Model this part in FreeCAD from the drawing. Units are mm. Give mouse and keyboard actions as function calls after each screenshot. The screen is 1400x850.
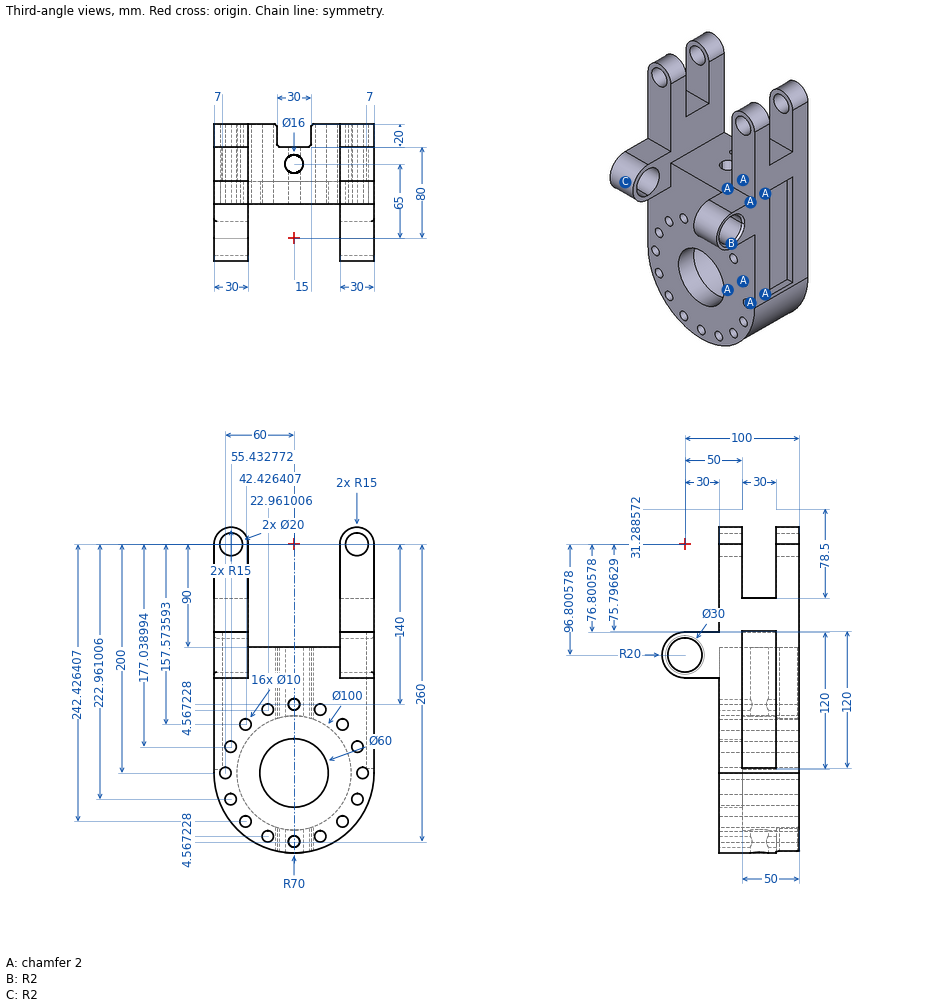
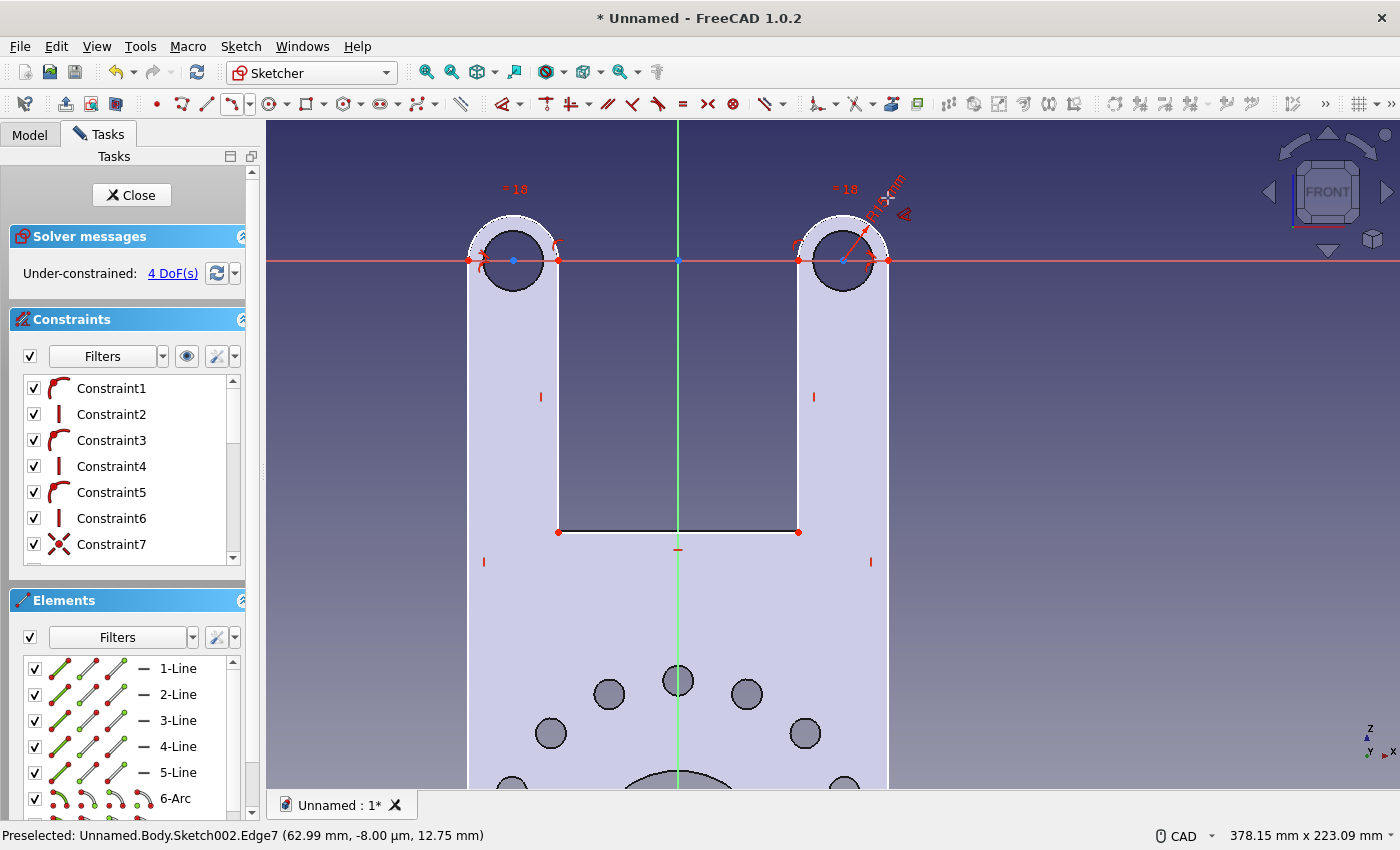
click(798, 342)
click(832, 397)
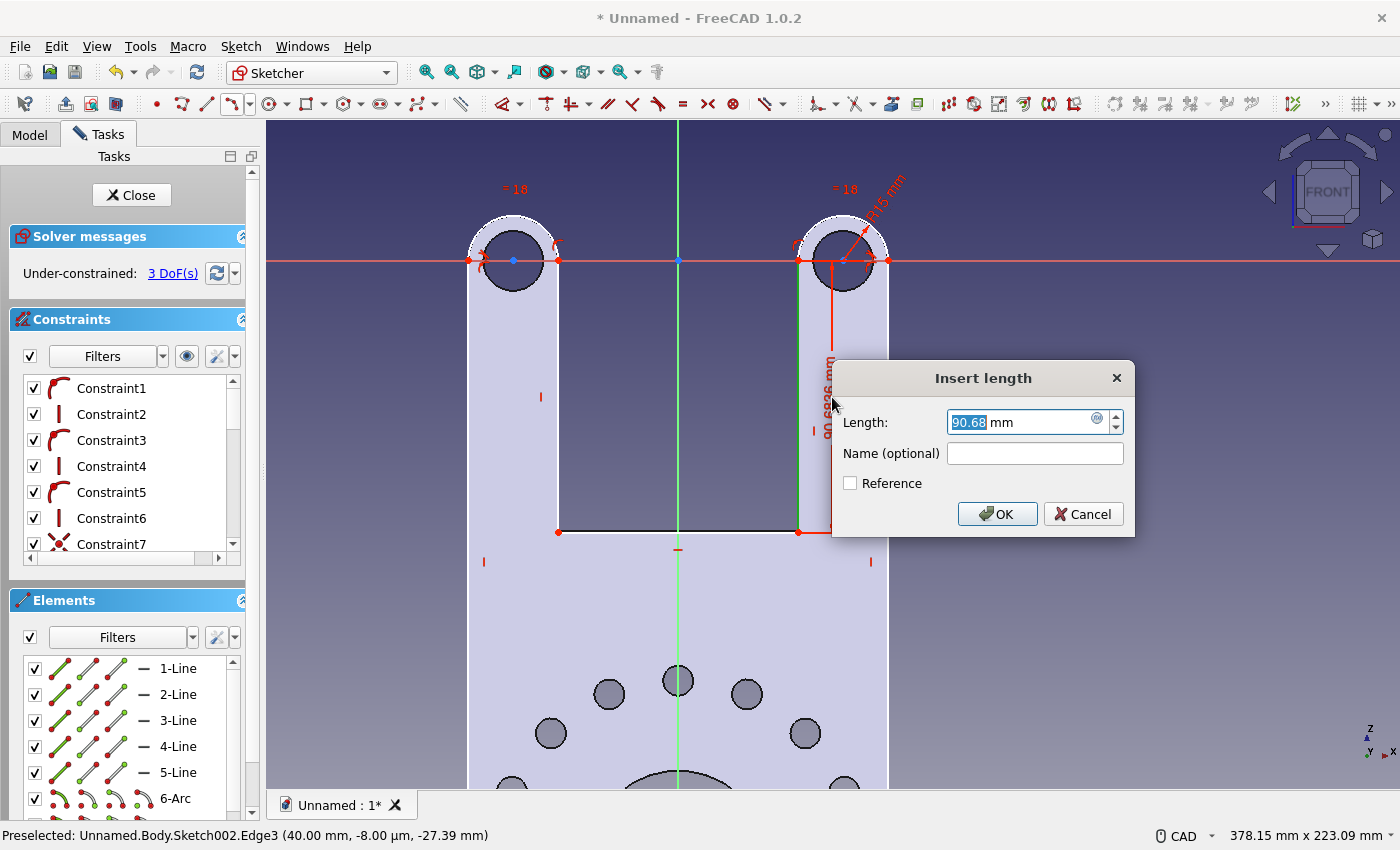
text(90)
key(Return)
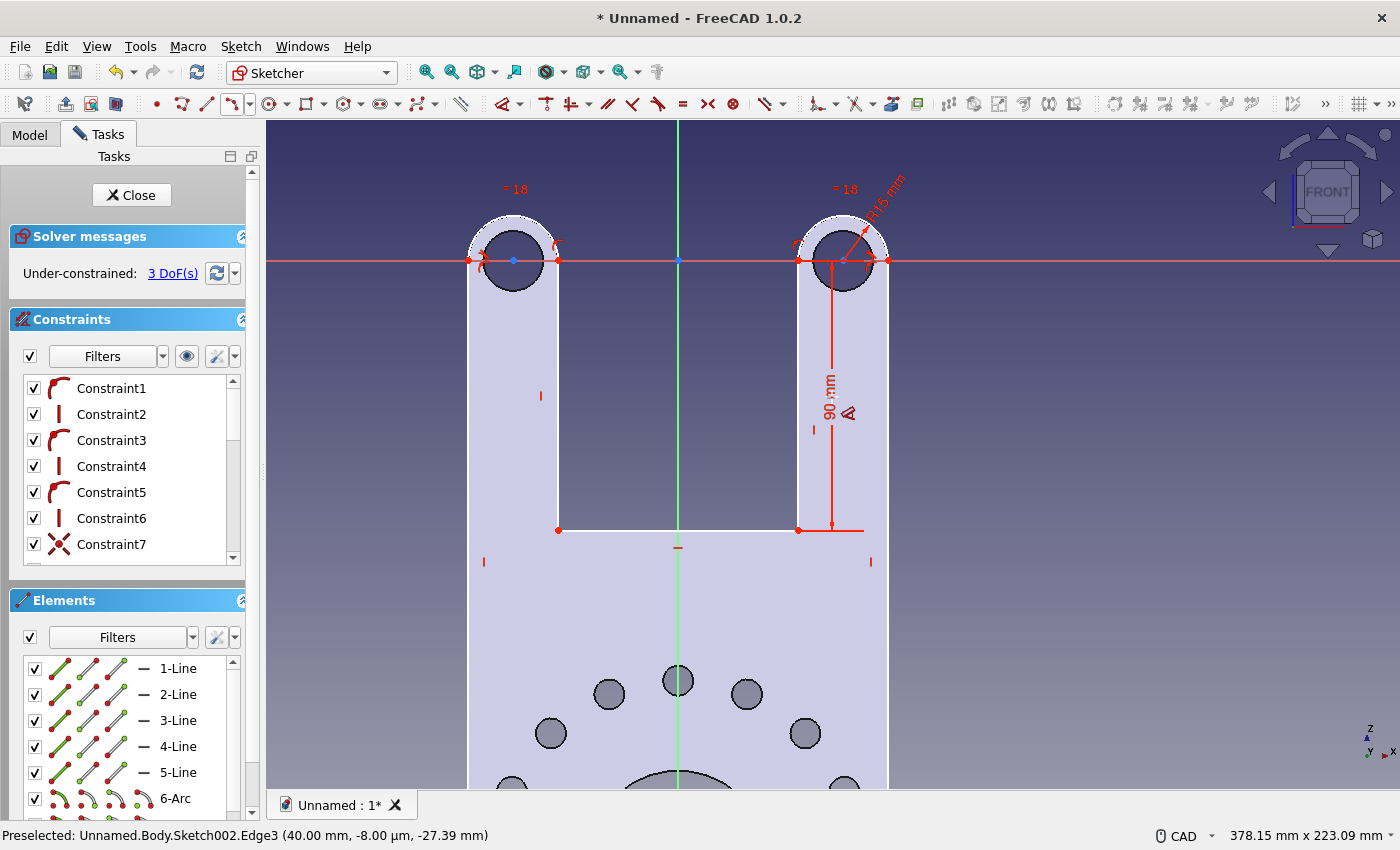
click(468, 441)
click(434, 511)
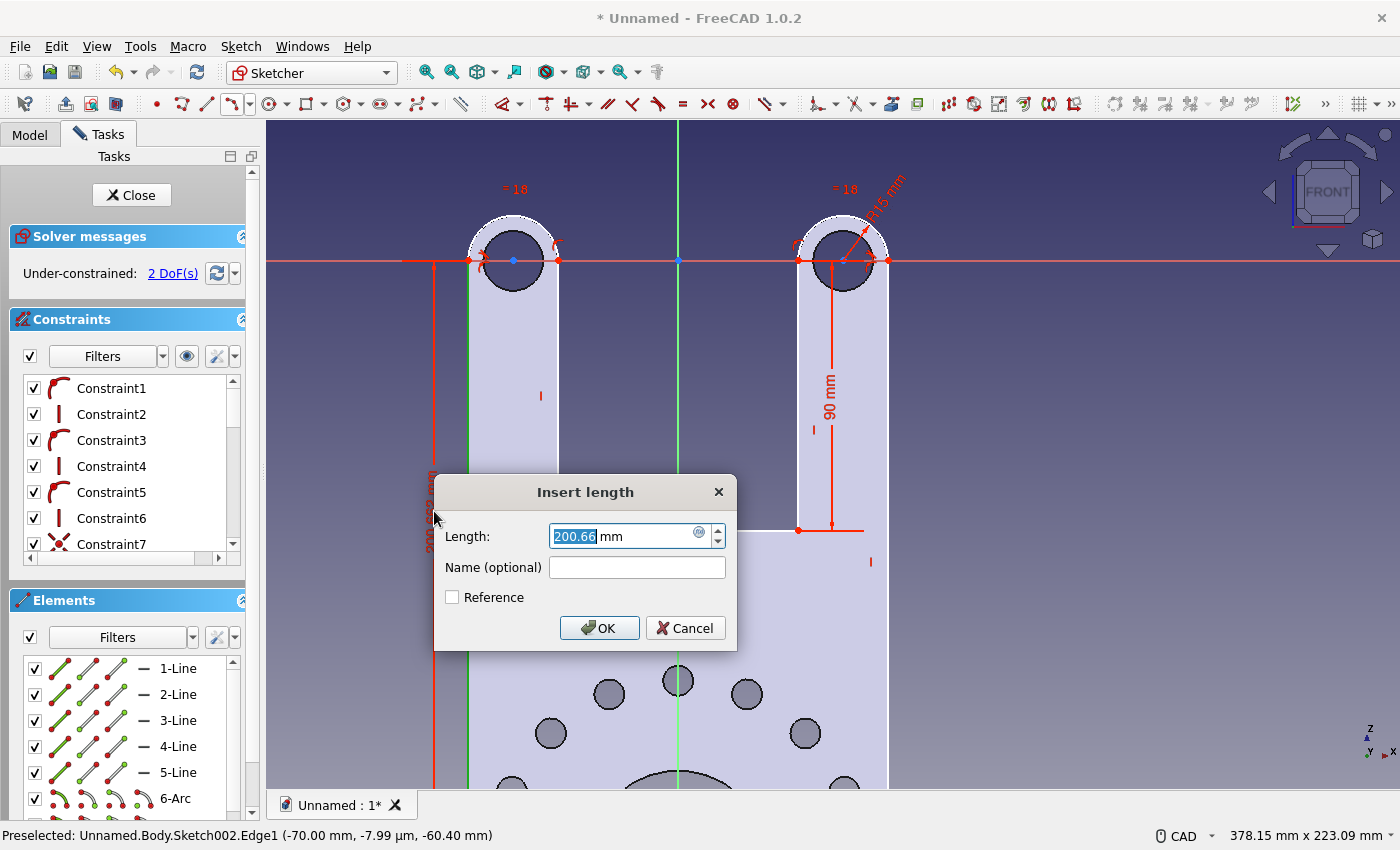
text(200)
key(Return)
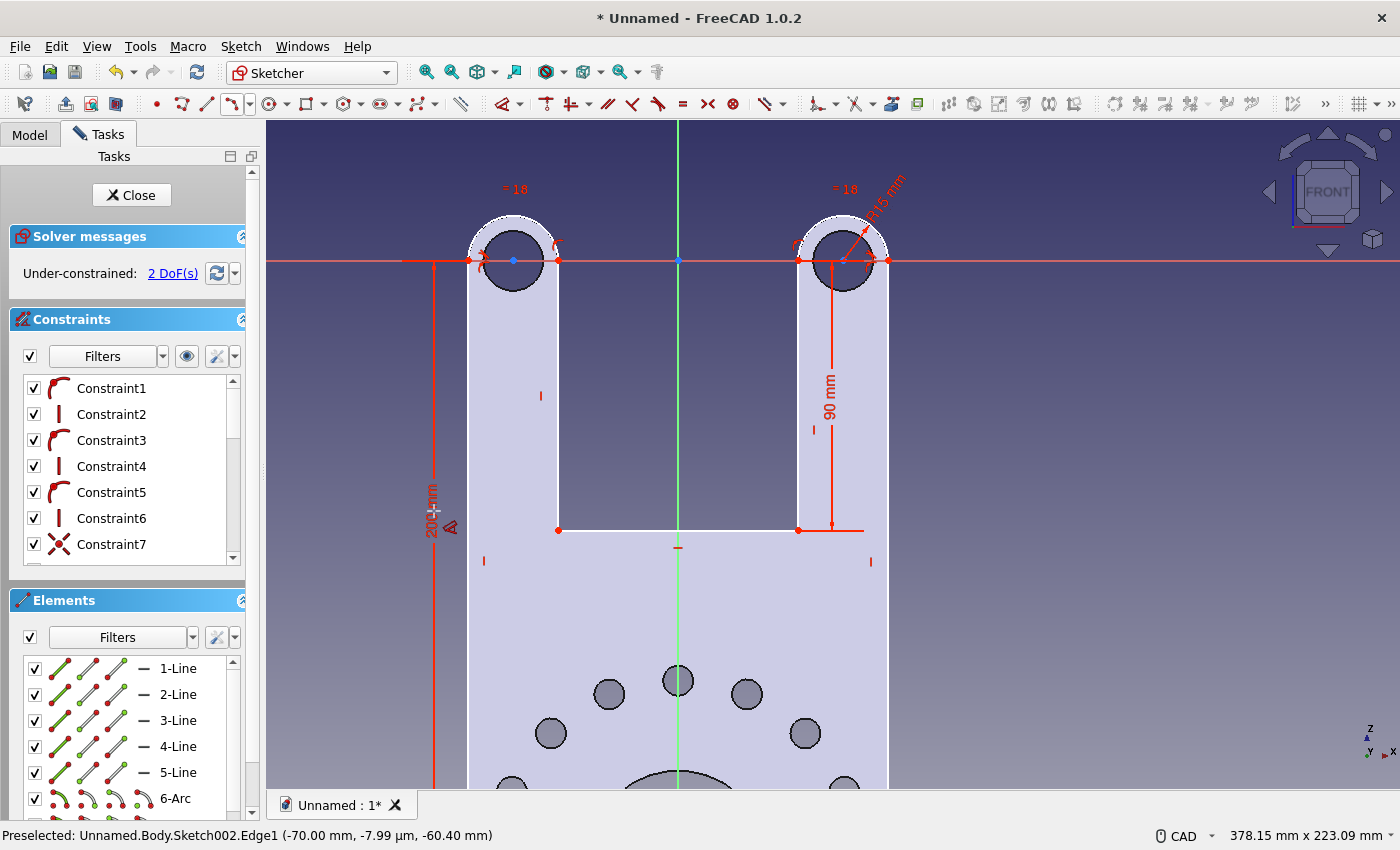
click(888, 682)
click(922, 511)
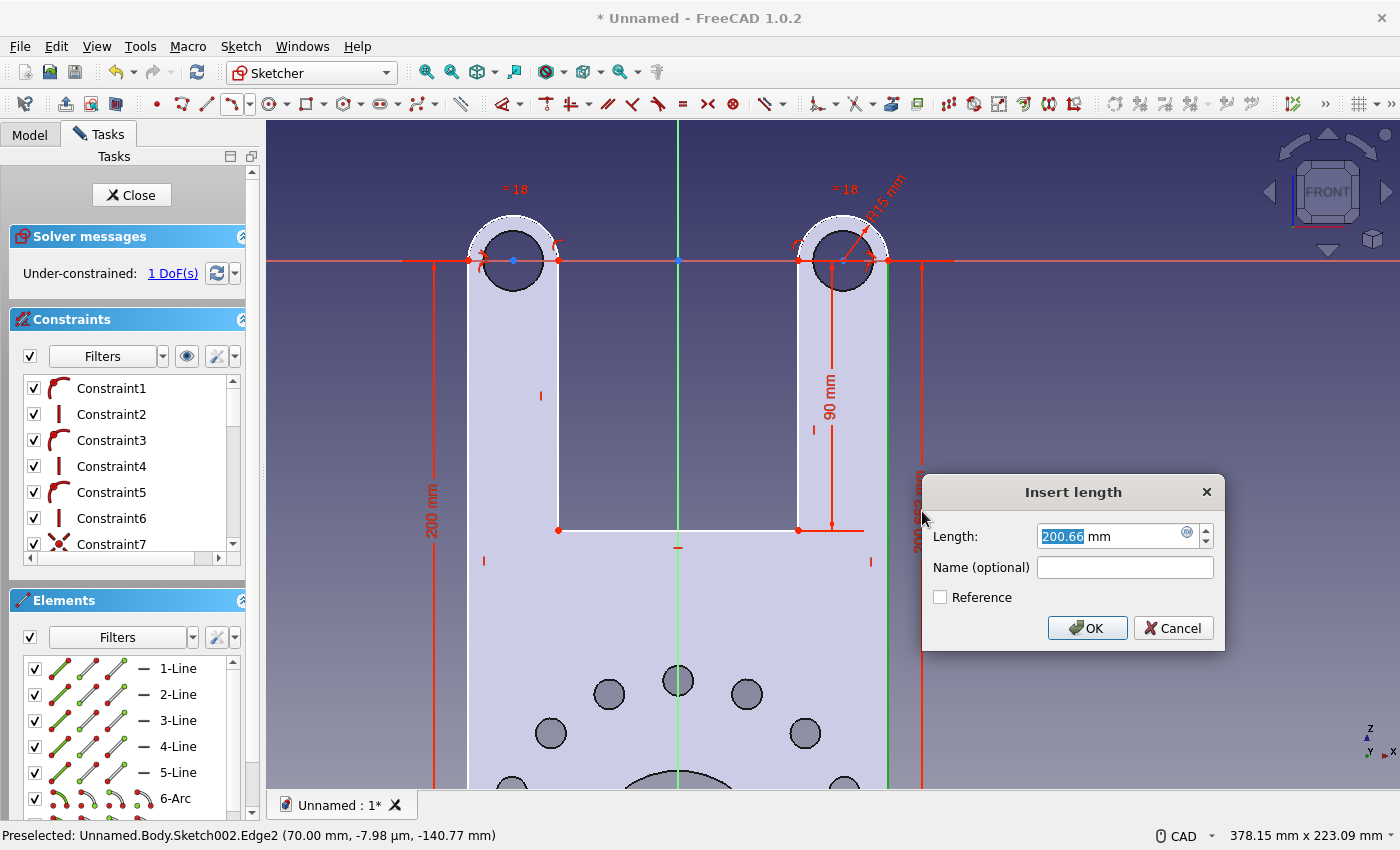
text(200)
key(Return)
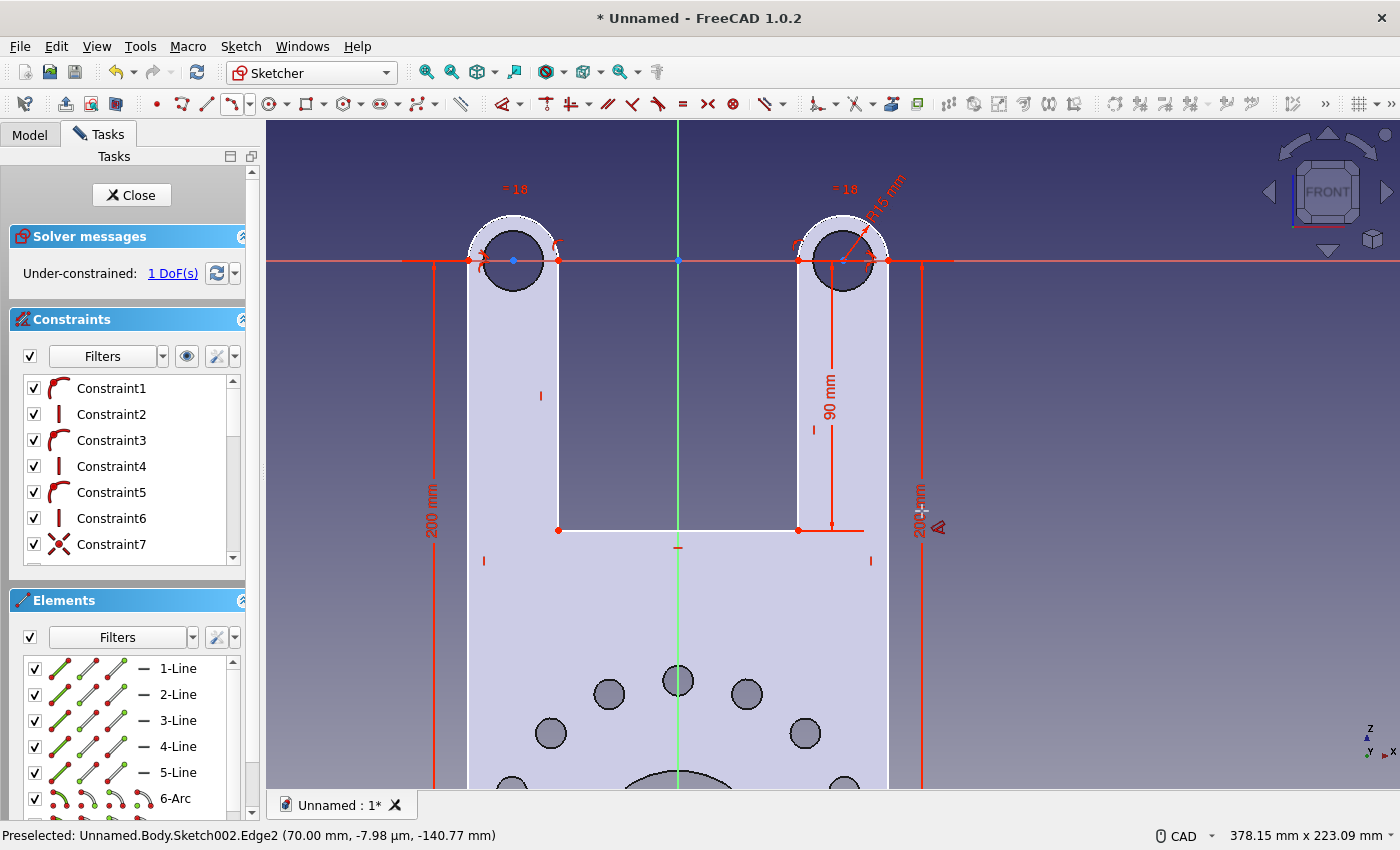
scroll(870, 225, down, 3)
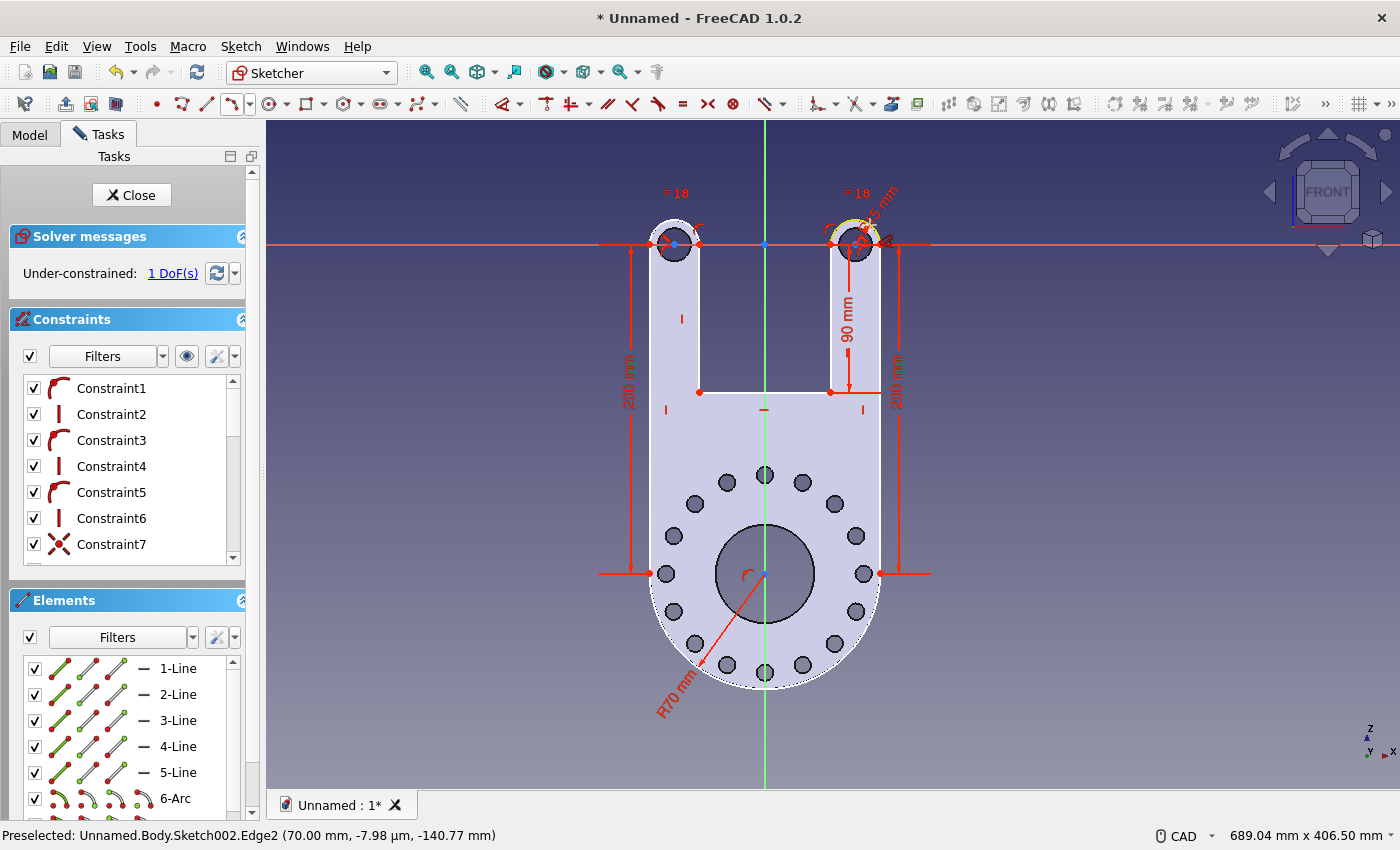
click(765, 574)
click(799, 409)